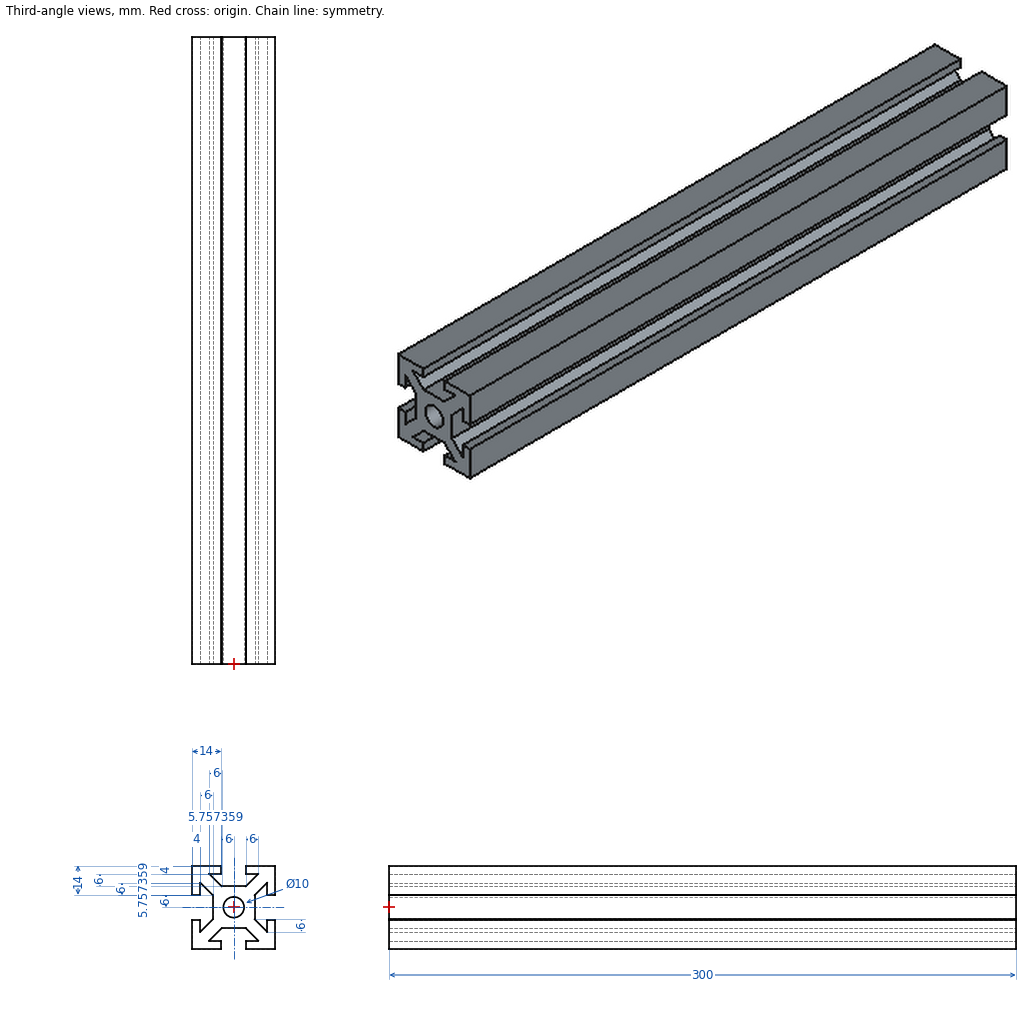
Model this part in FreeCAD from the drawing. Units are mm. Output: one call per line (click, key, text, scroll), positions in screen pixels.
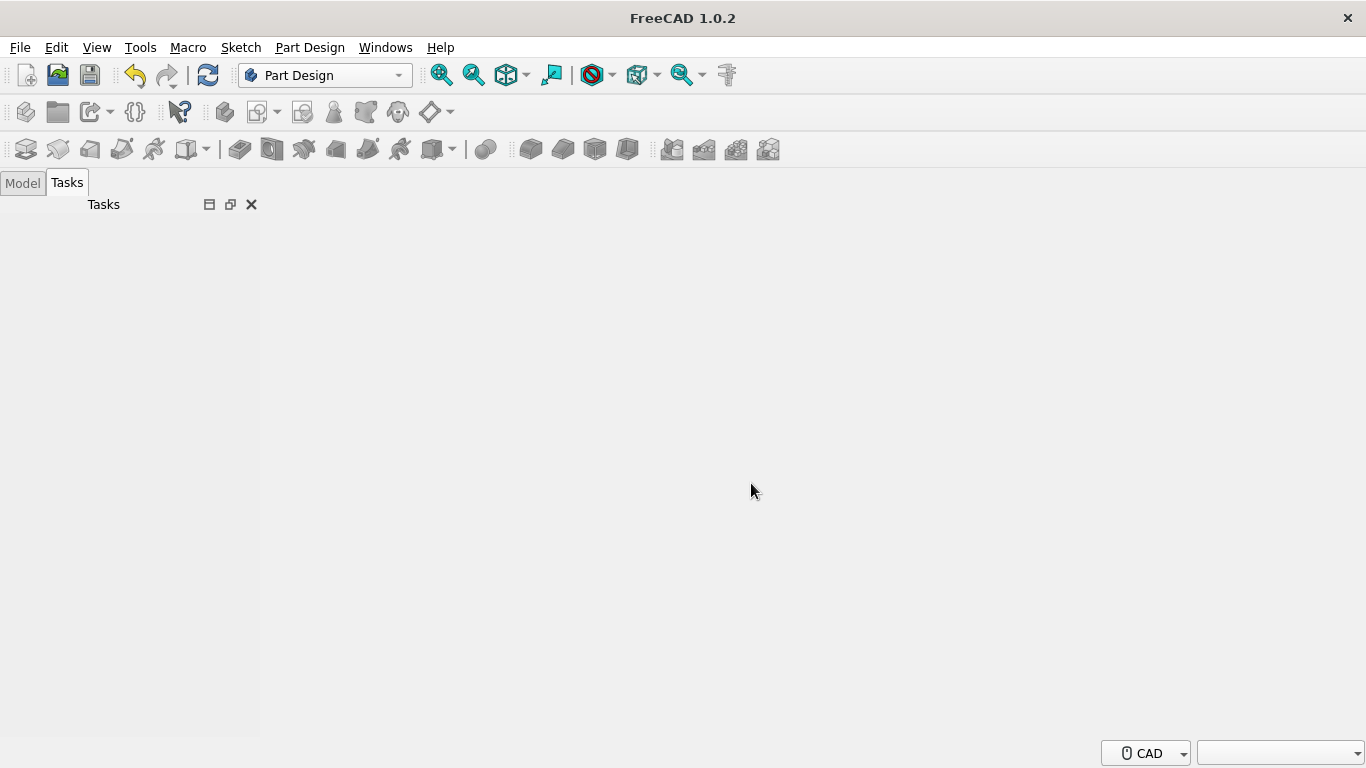
click(26, 76)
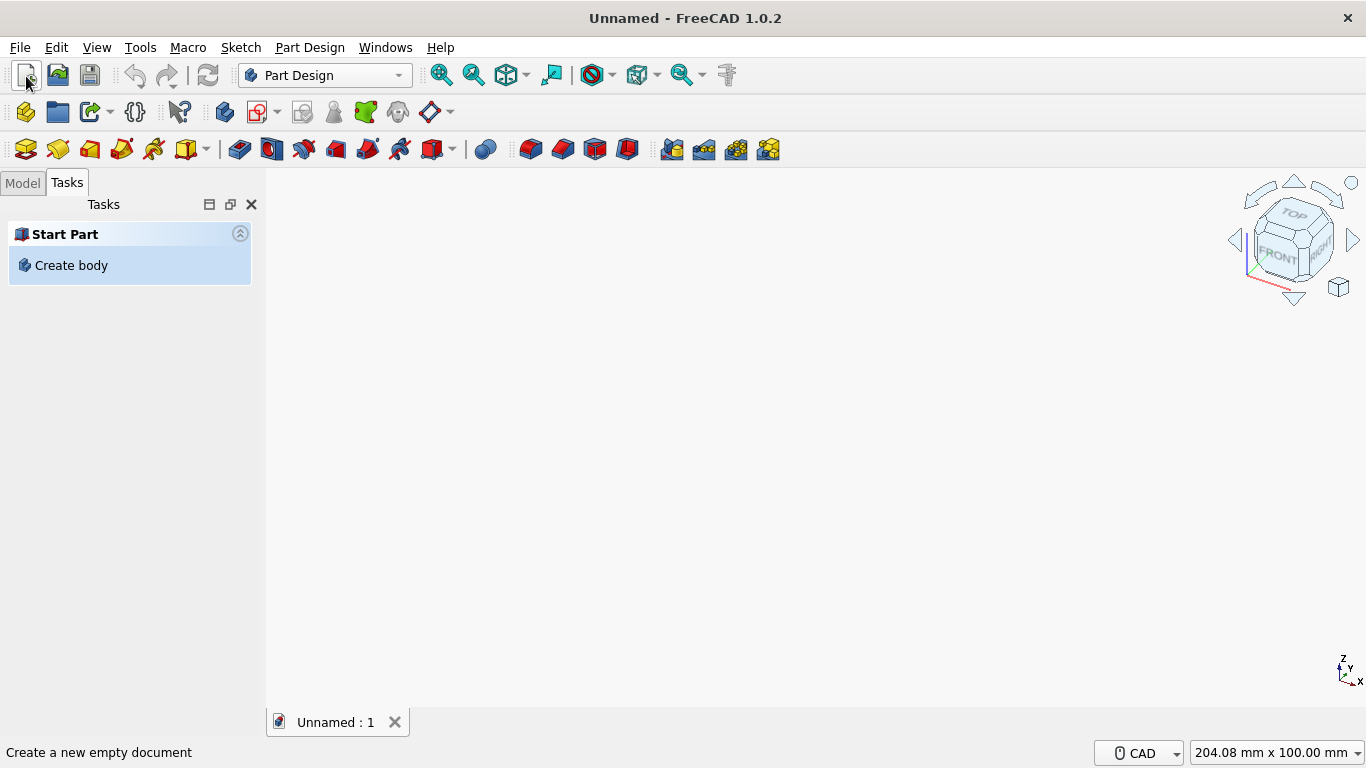
click(258, 112)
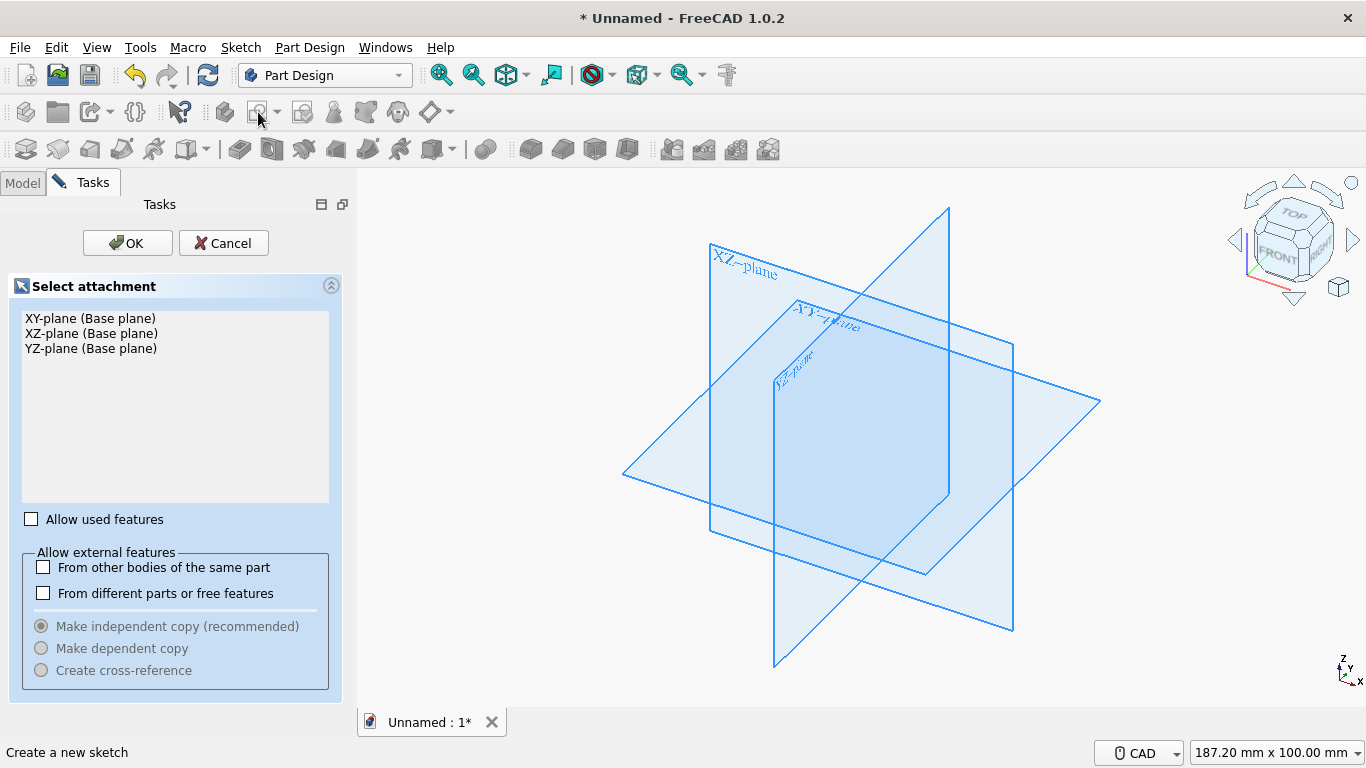
click(82, 334)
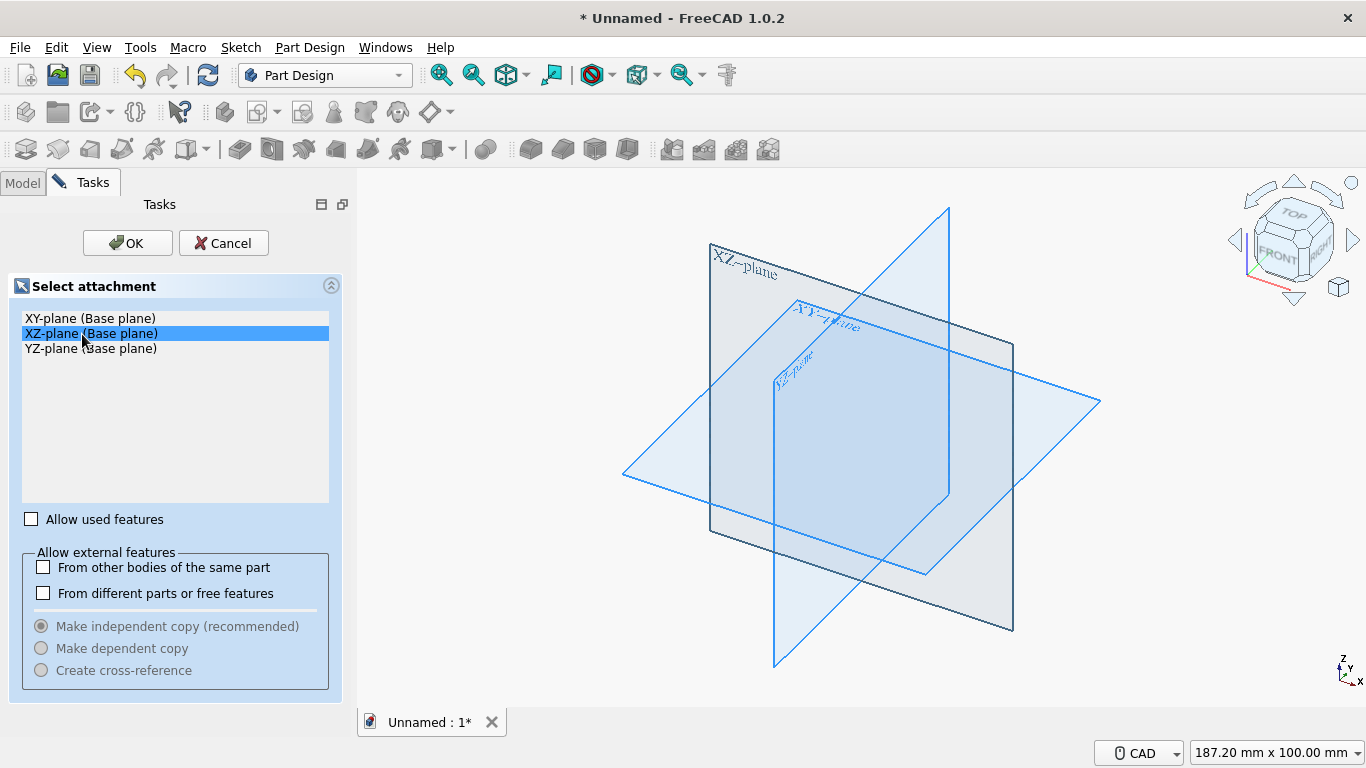
click(128, 243)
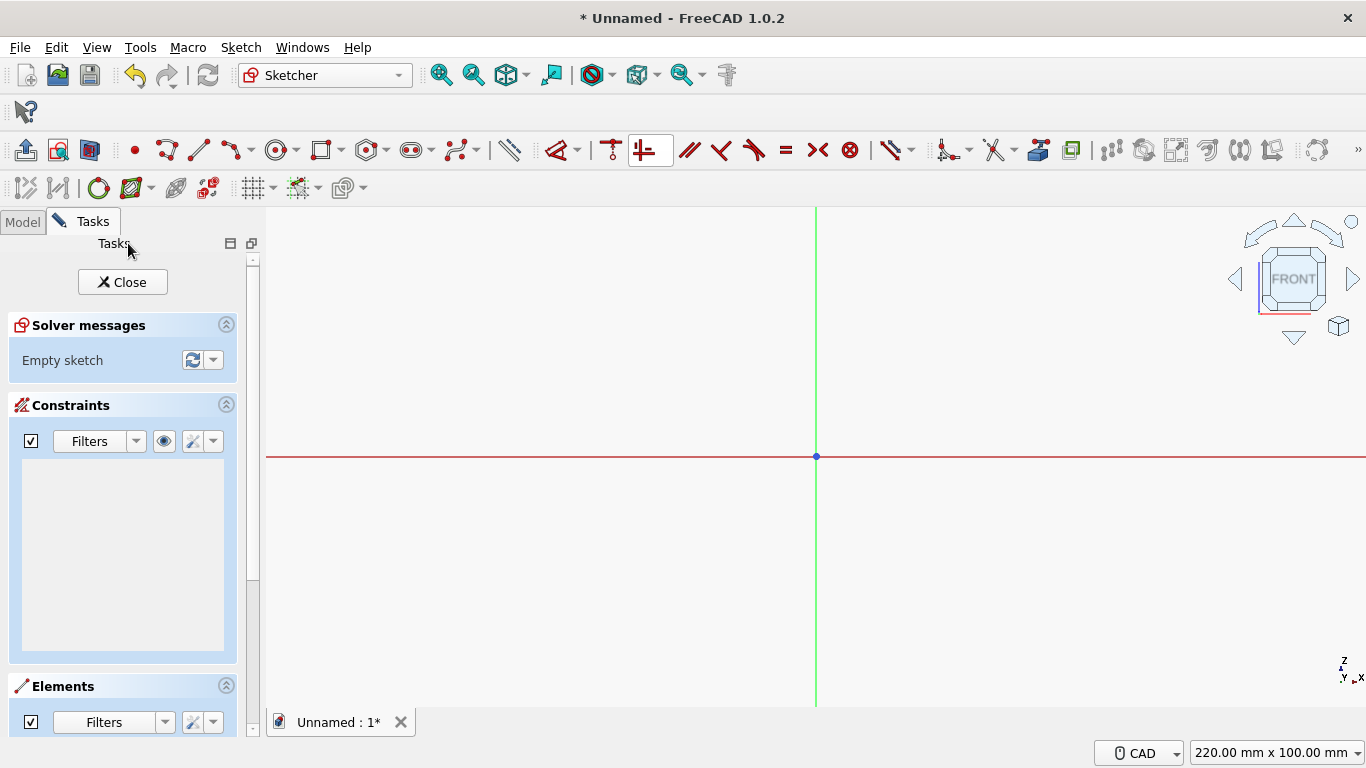
scroll(955, 457, up, 2)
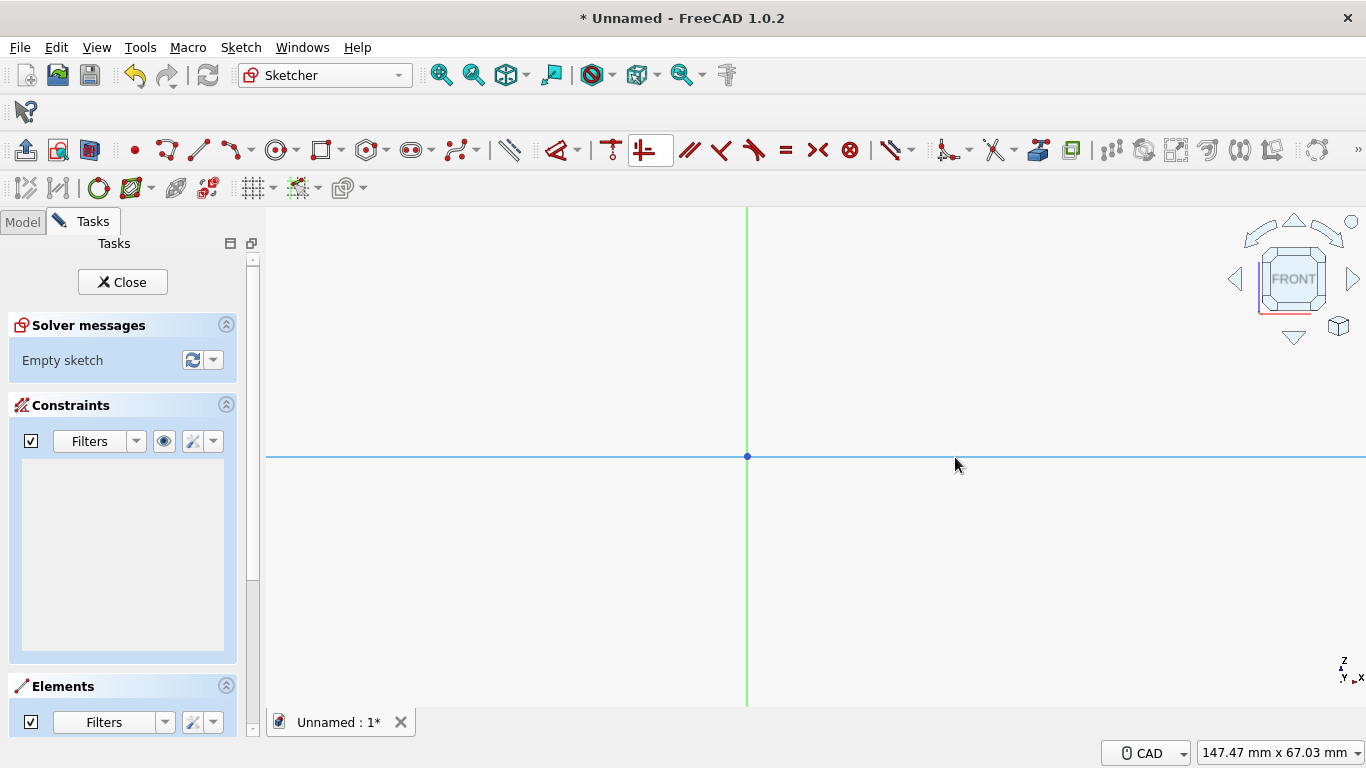
click(168, 150)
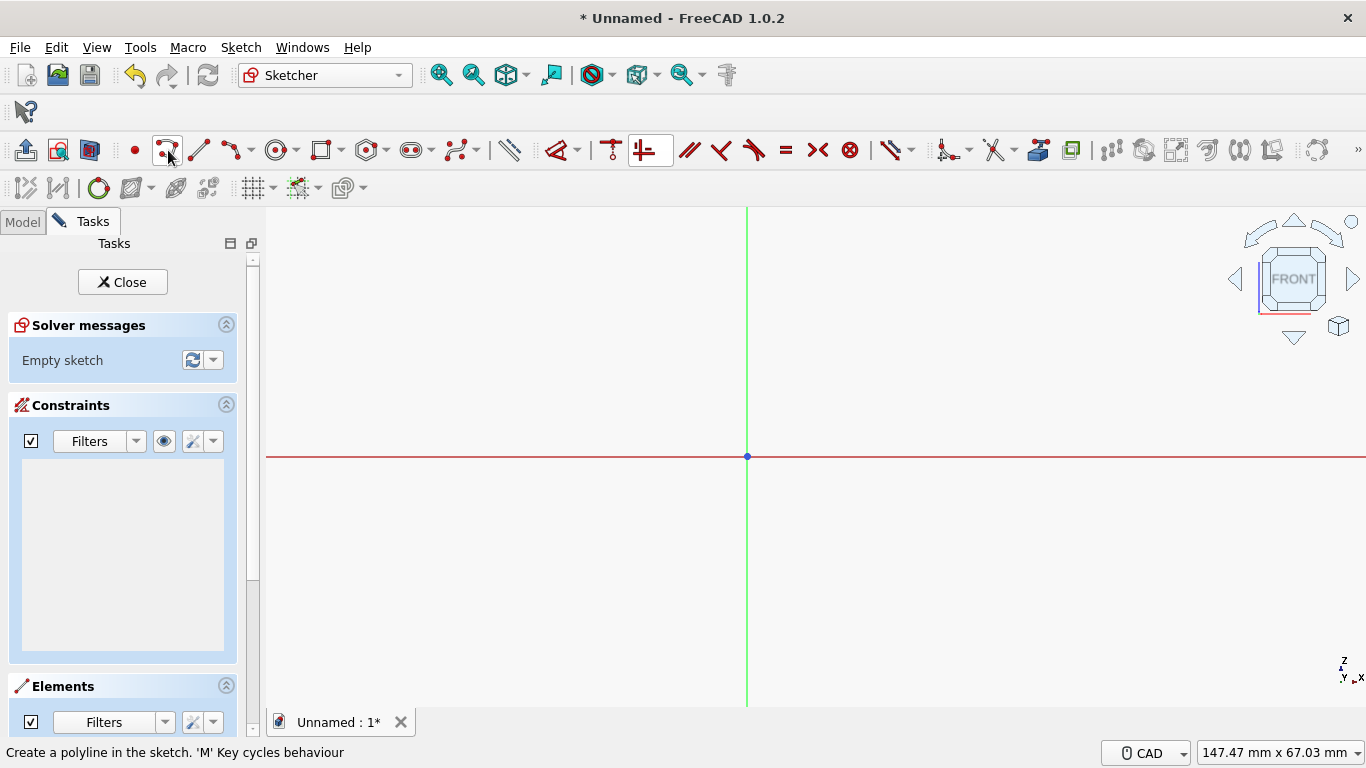
click(673, 500)
click(673, 414)
click(628, 369)
click(628, 412)
click(598, 412)
click(598, 308)
click(703, 308)
click(703, 337)
click(660, 337)
click(704, 382)
click(790, 382)
click(835, 337)
click(792, 337)
click(792, 308)
click(897, 308)
click(897, 412)
click(867, 412)
click(867, 369)
click(822, 414)
click(822, 500)
click(867, 544)
click(867, 502)
click(897, 502)
click(897, 606)
click(792, 606)
click(792, 576)
click(835, 576)
click(790, 531)
click(704, 531)
click(660, 576)
click(703, 576)
click(703, 606)
click(598, 606)
click(598, 502)
click(628, 502)
click(628, 544)
click(673, 501)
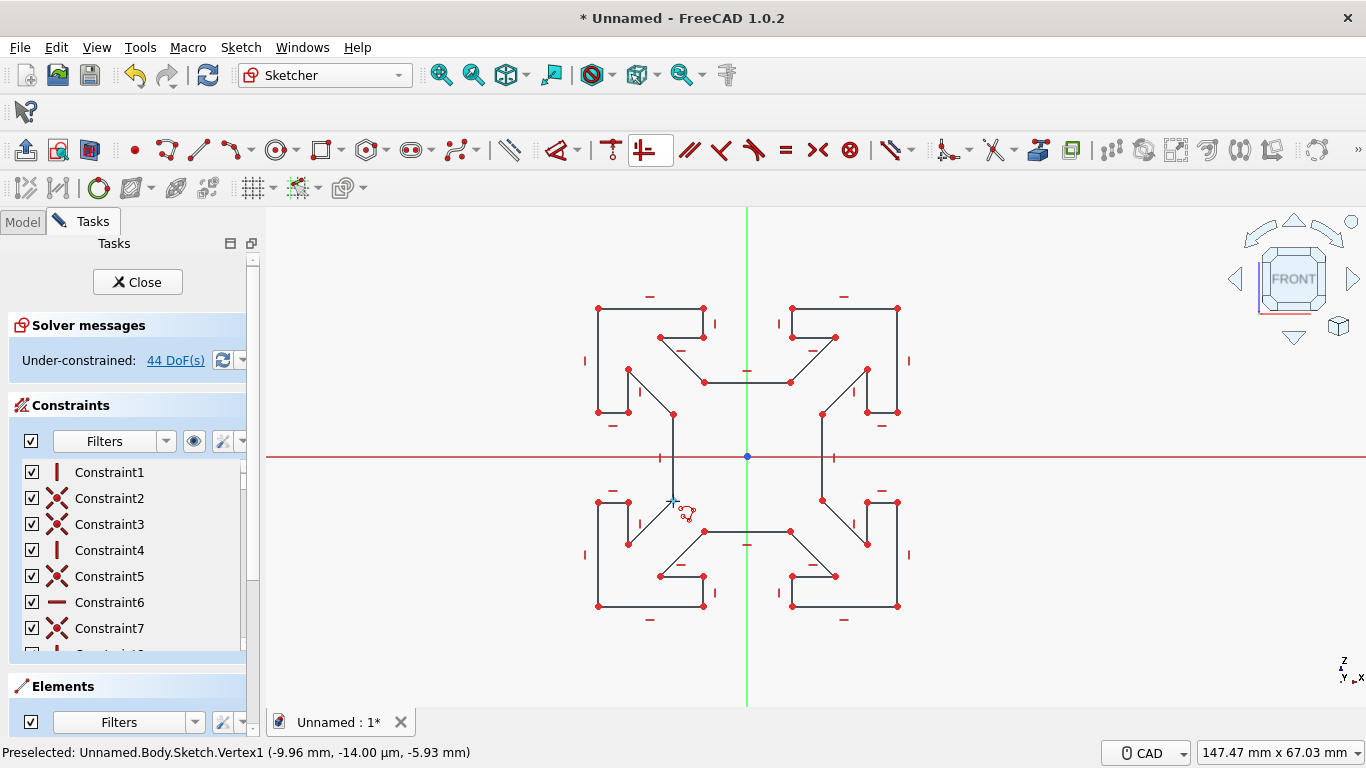
click(276, 150)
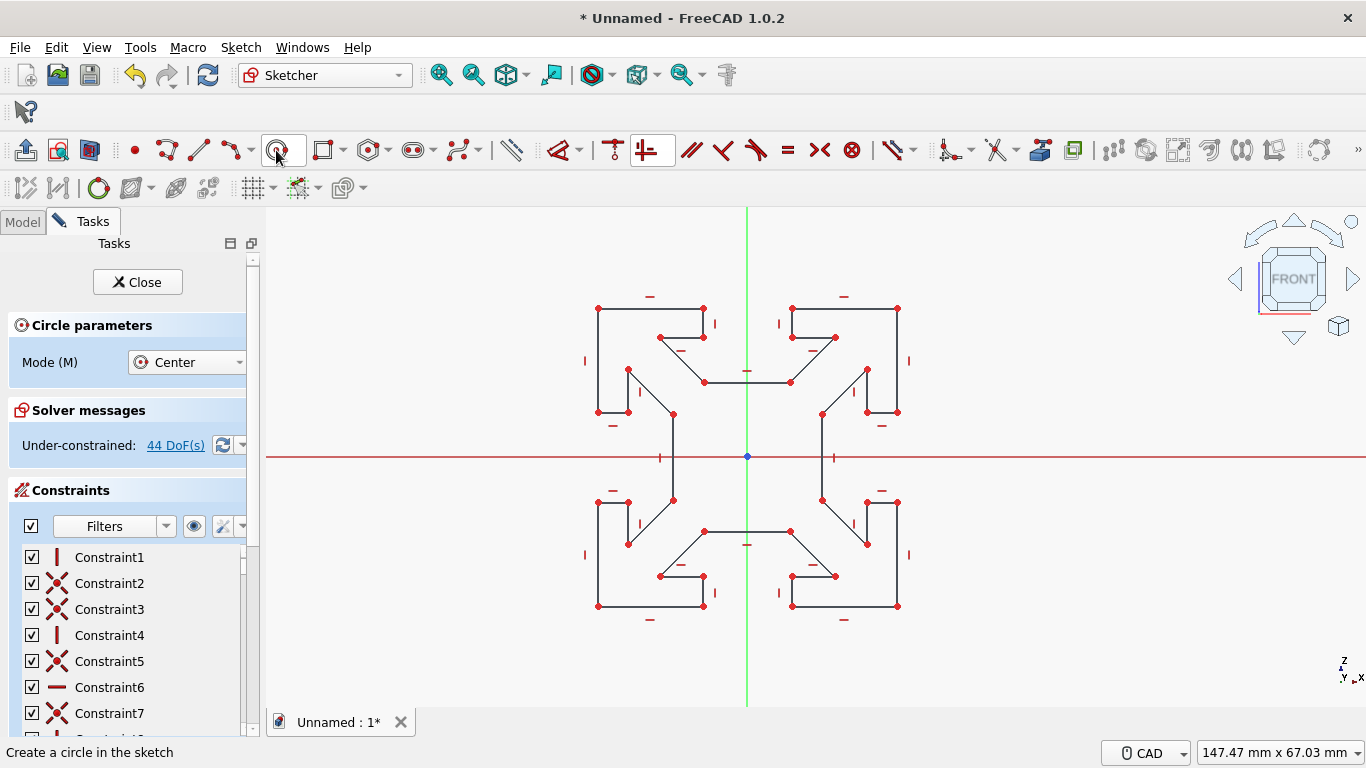
click(747, 457)
click(774, 430)
key(Escape)